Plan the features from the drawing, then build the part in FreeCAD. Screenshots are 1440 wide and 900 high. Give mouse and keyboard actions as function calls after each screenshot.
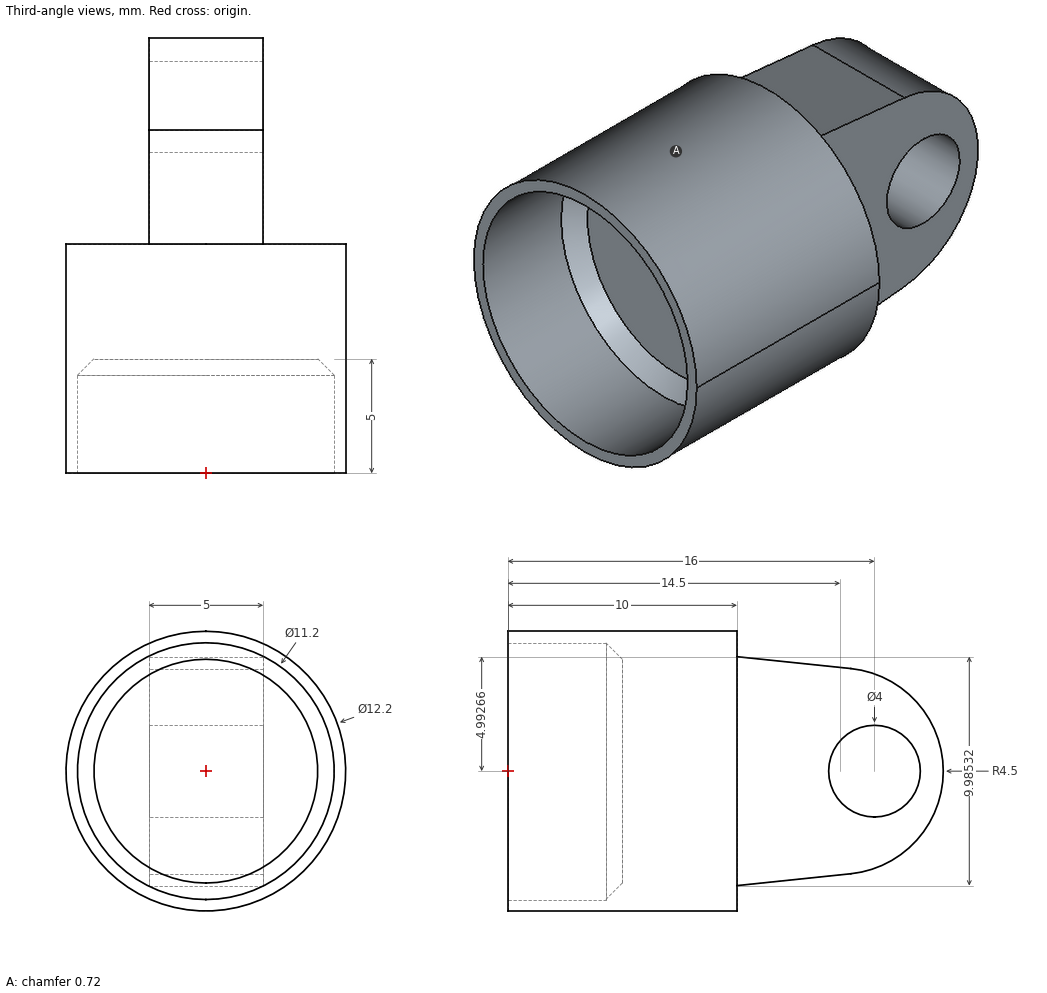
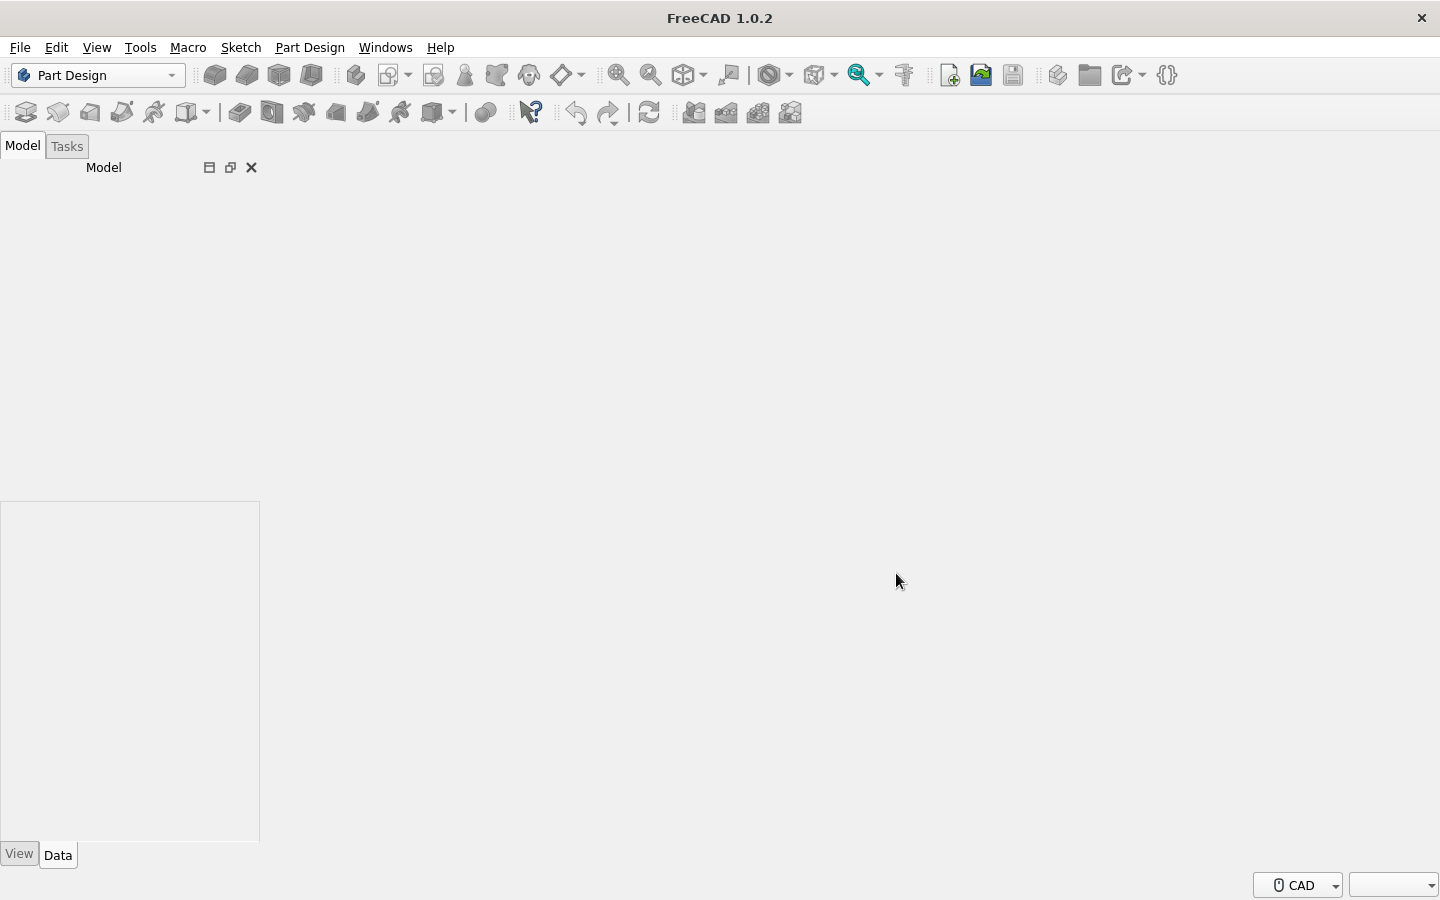
key(ctrl+n)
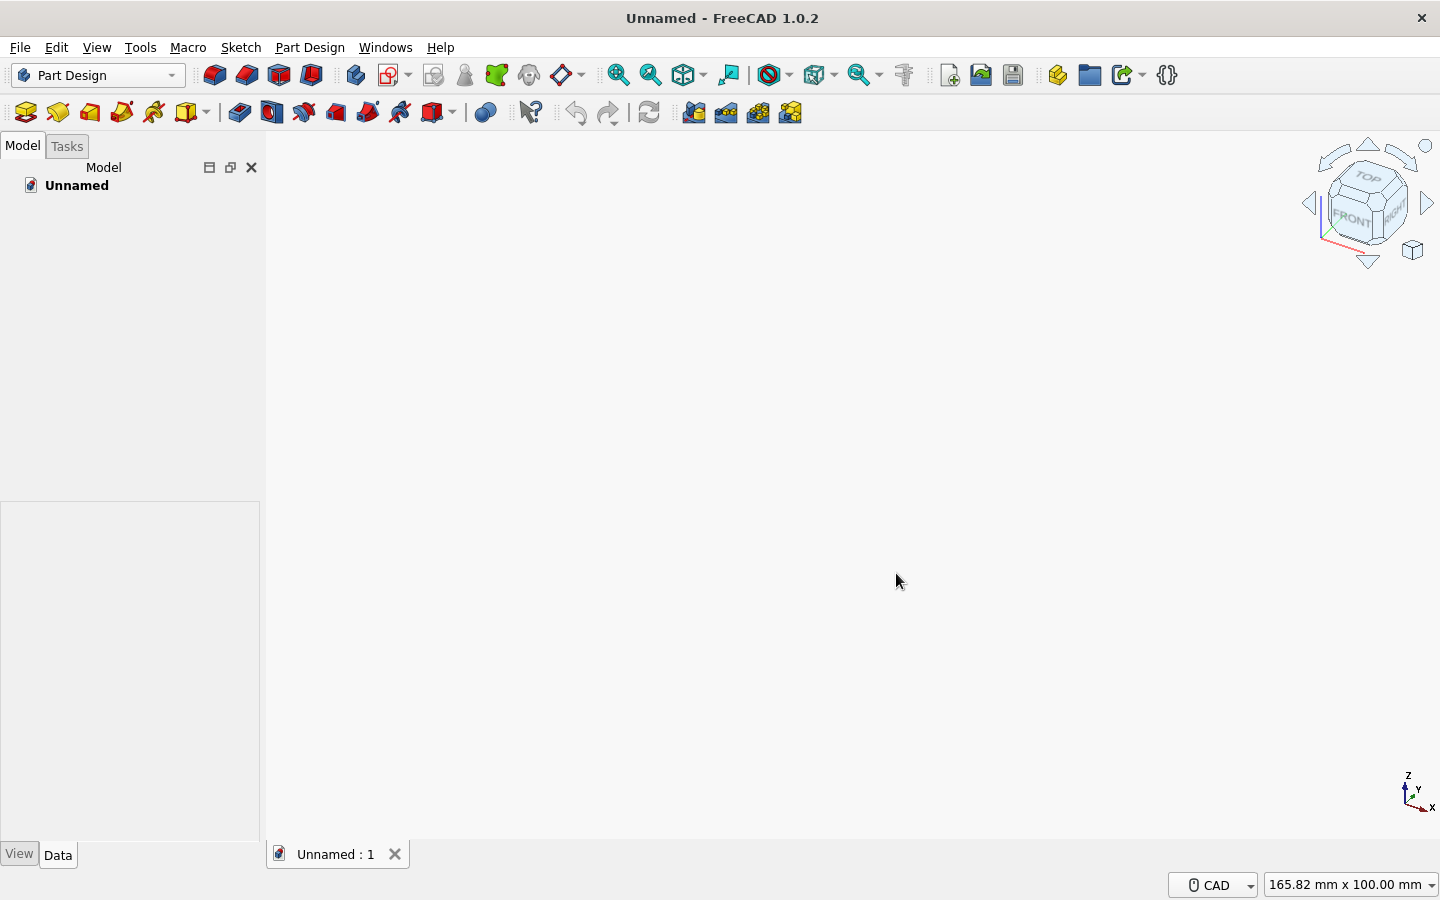
click(388, 76)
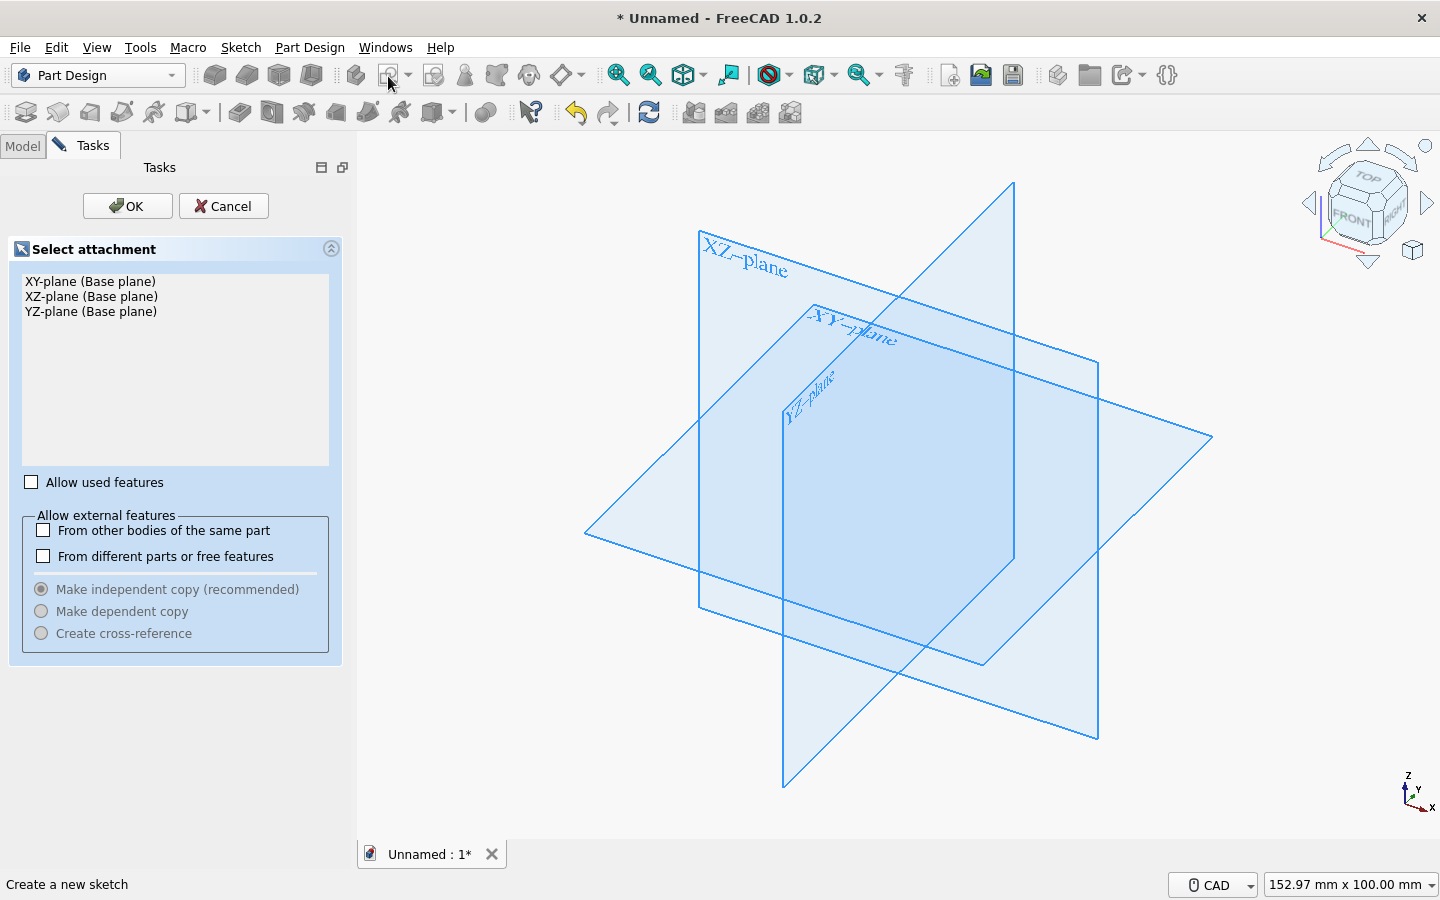
click(82, 296)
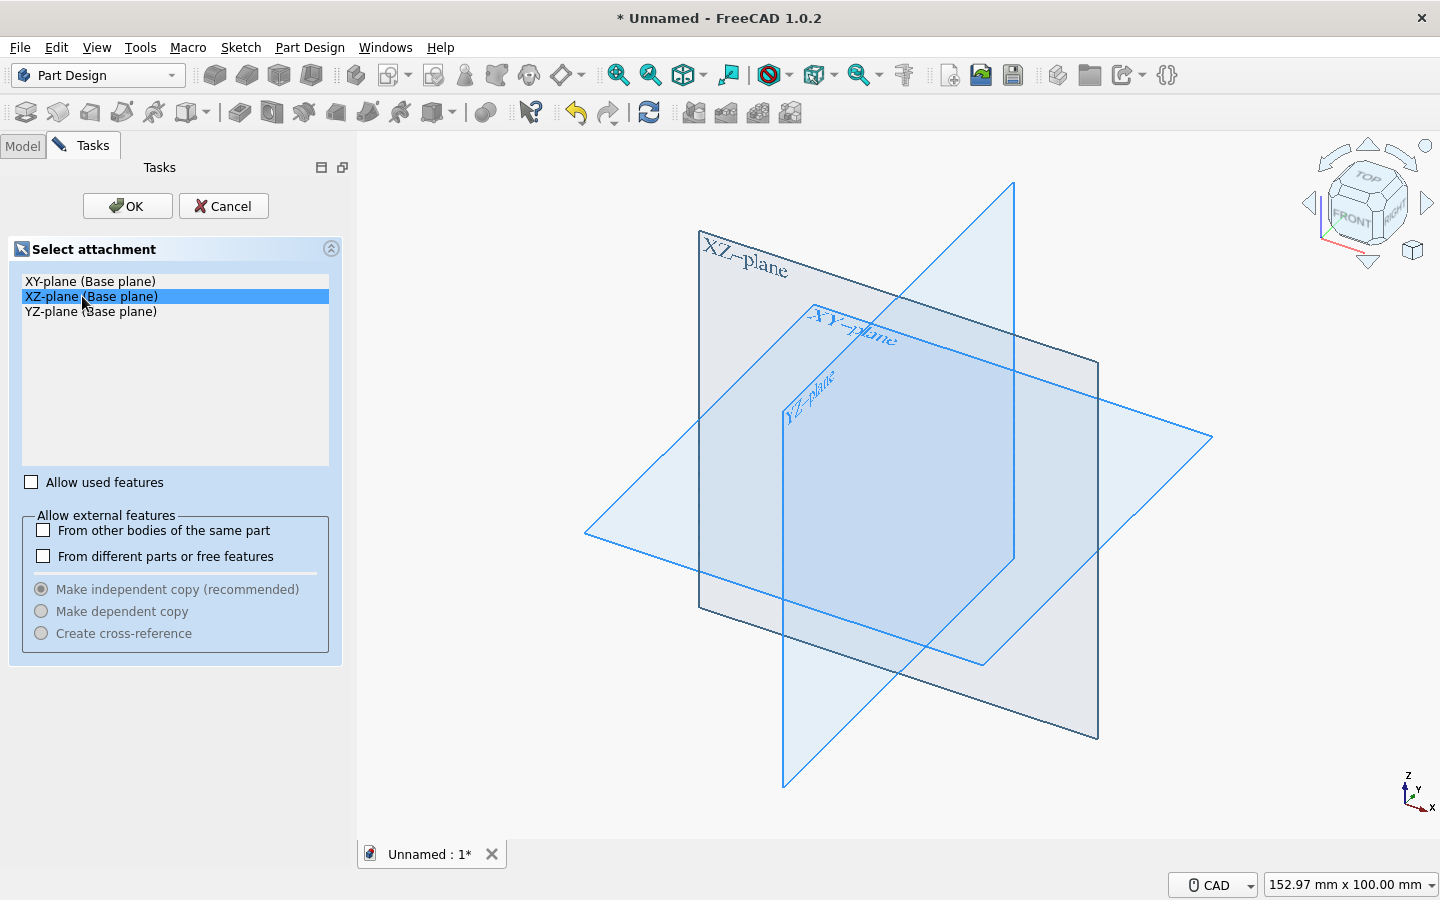
click(128, 206)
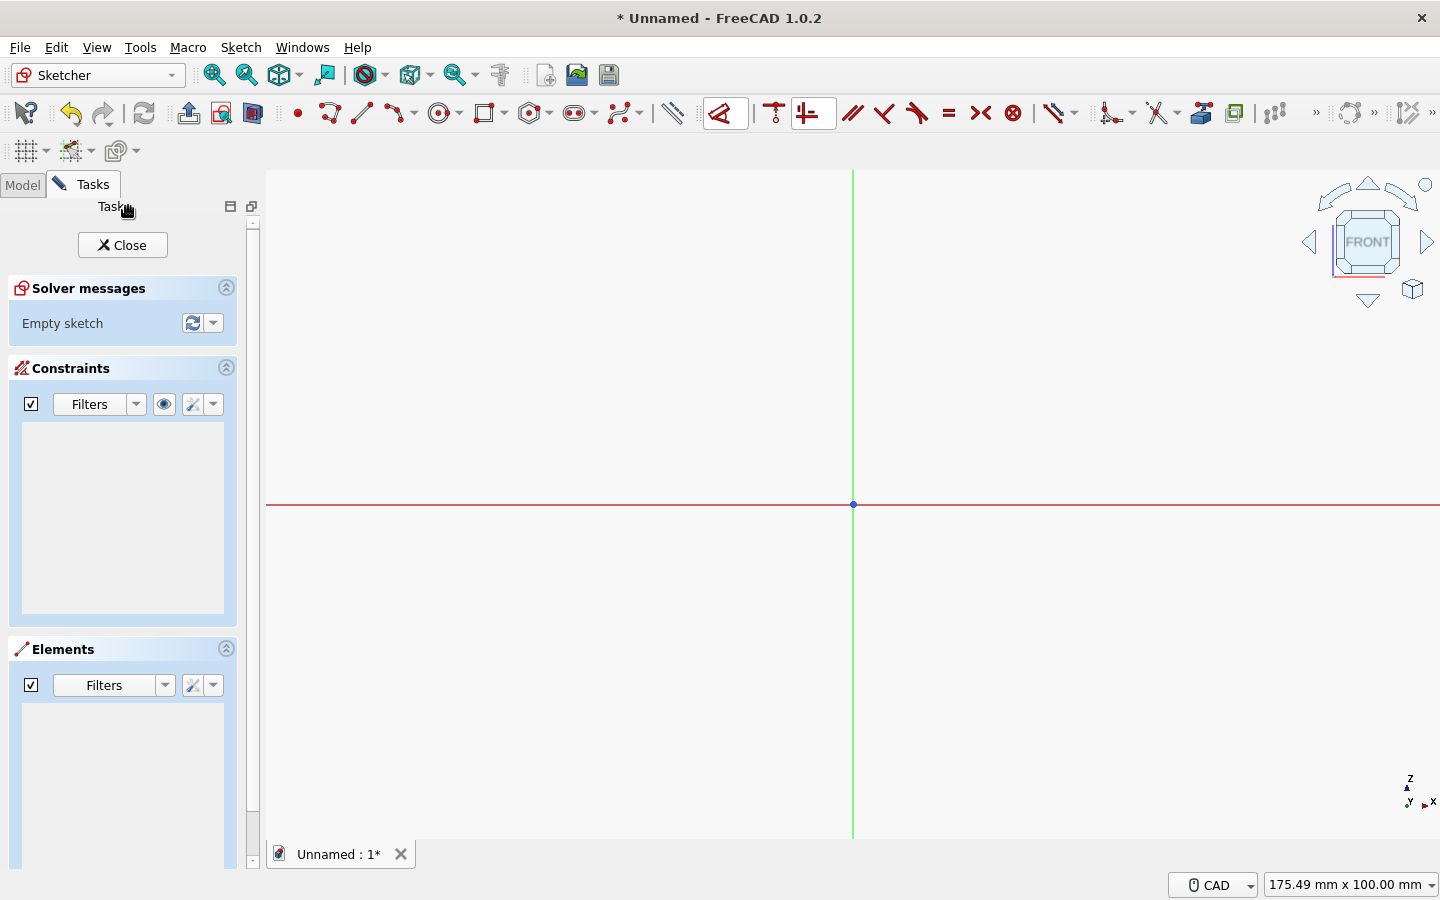
scroll(870, 504, up, 8)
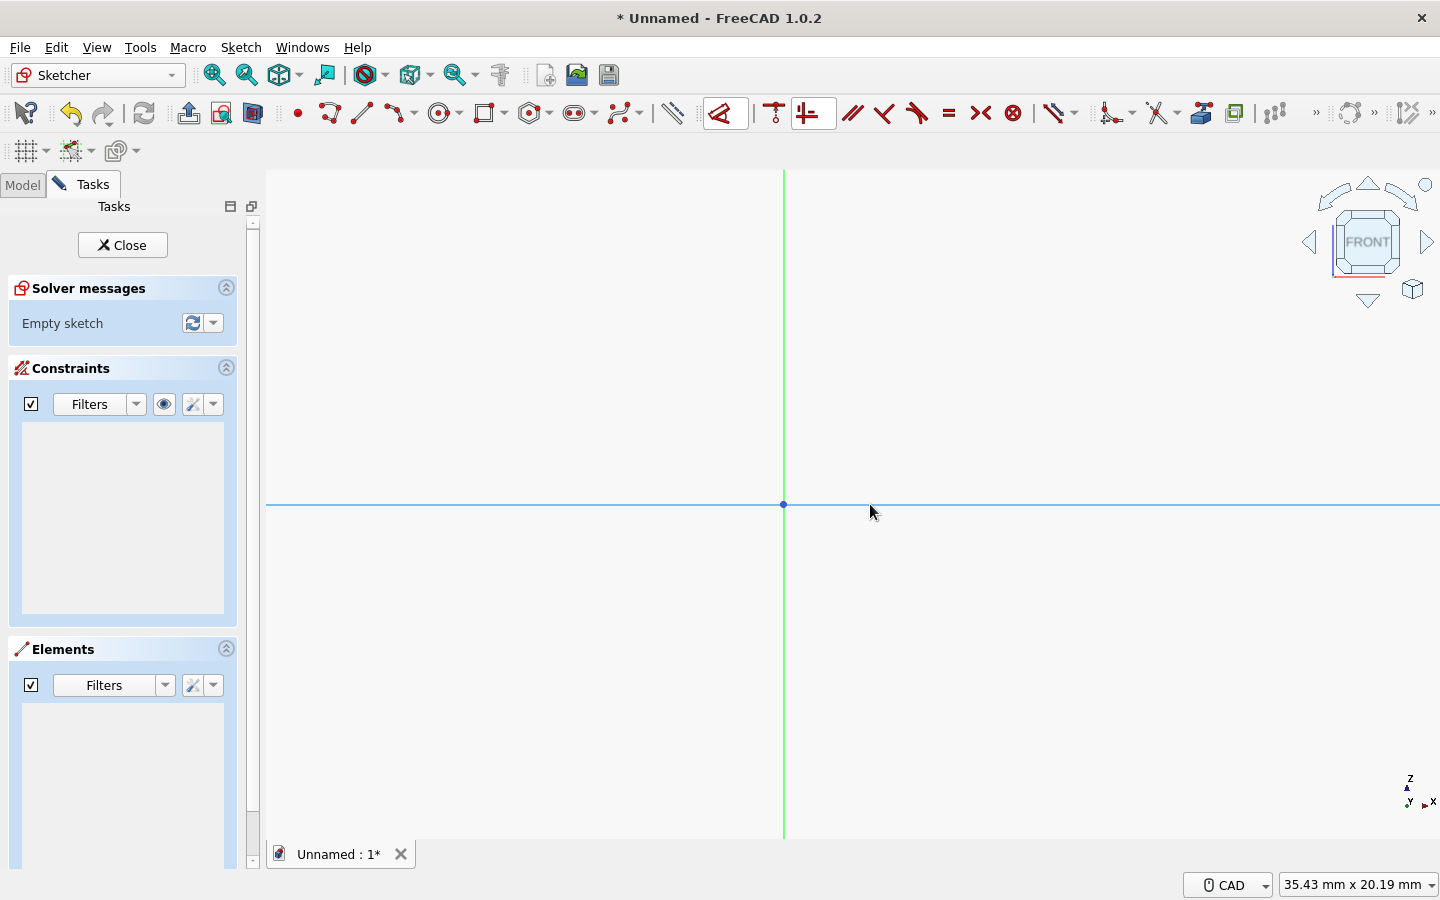
key(g)
key(c)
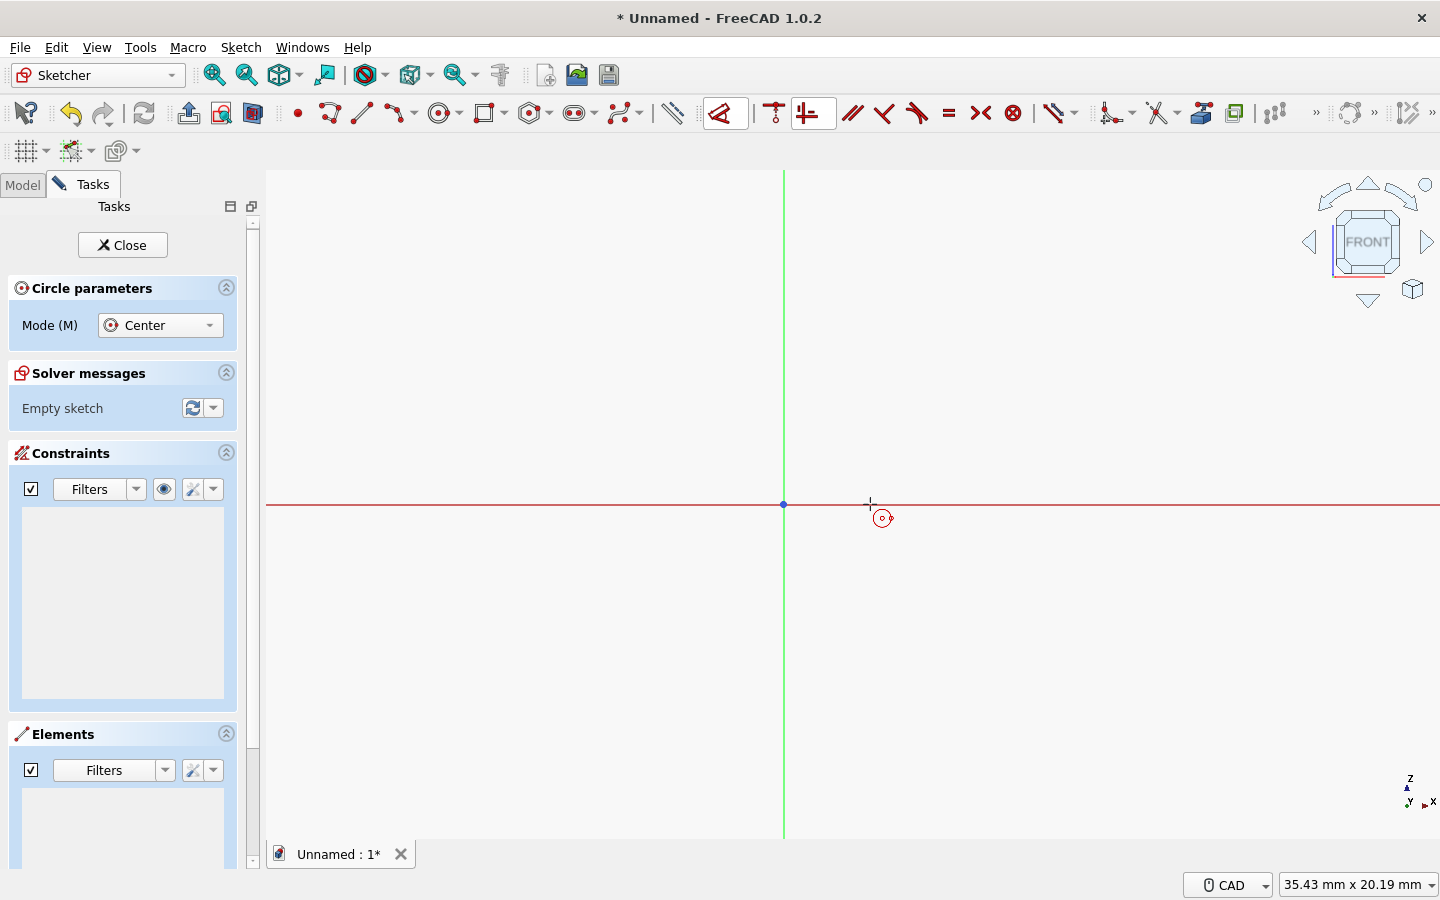
click(784, 504)
click(927, 362)
key(Escape)